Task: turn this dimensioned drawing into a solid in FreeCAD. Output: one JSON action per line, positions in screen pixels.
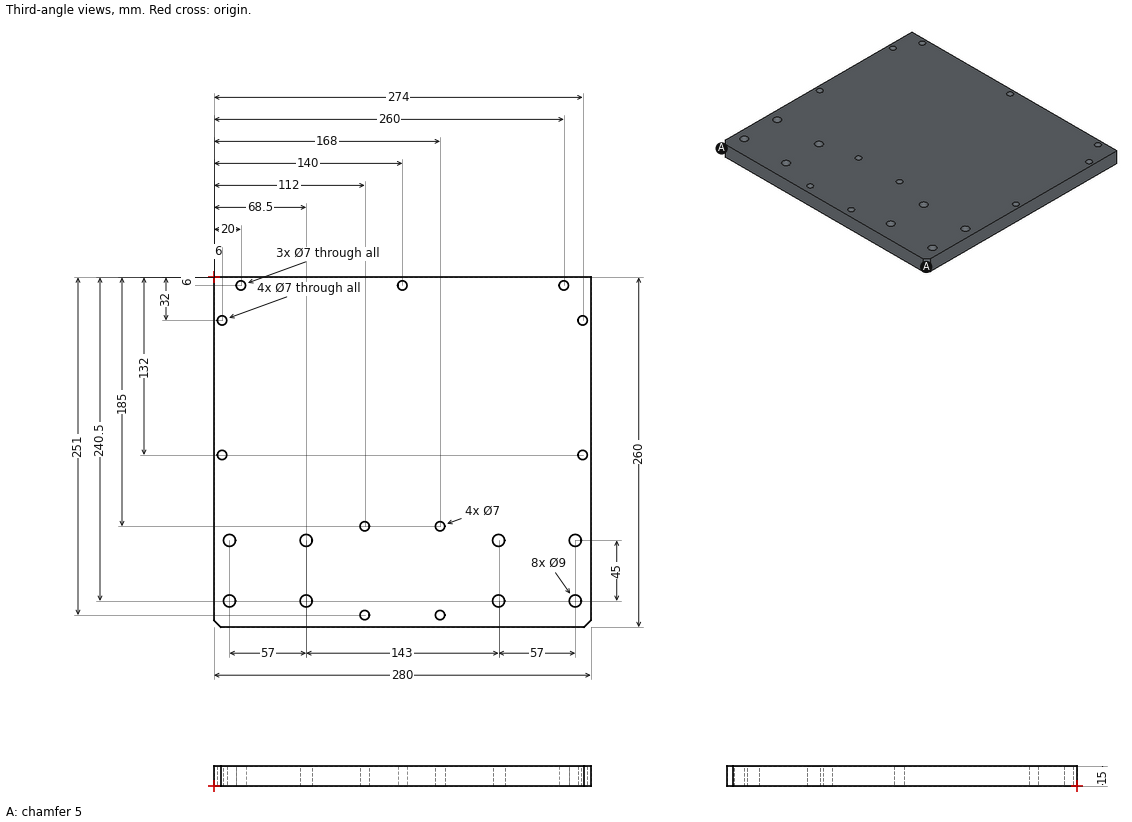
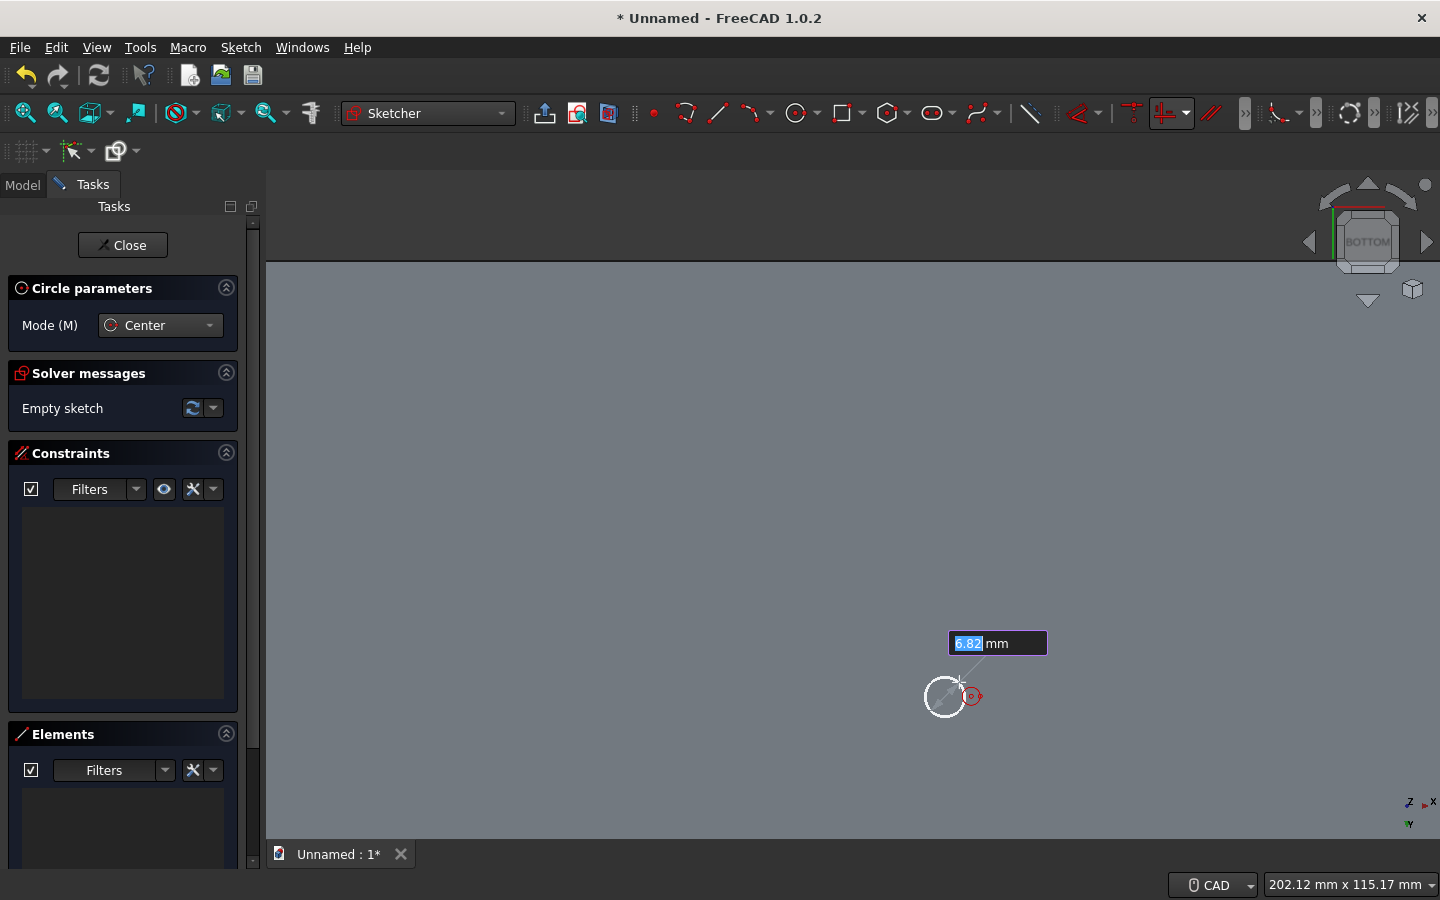
{"action": "type", "text": "7"}
{"action": "key", "text": "Return"}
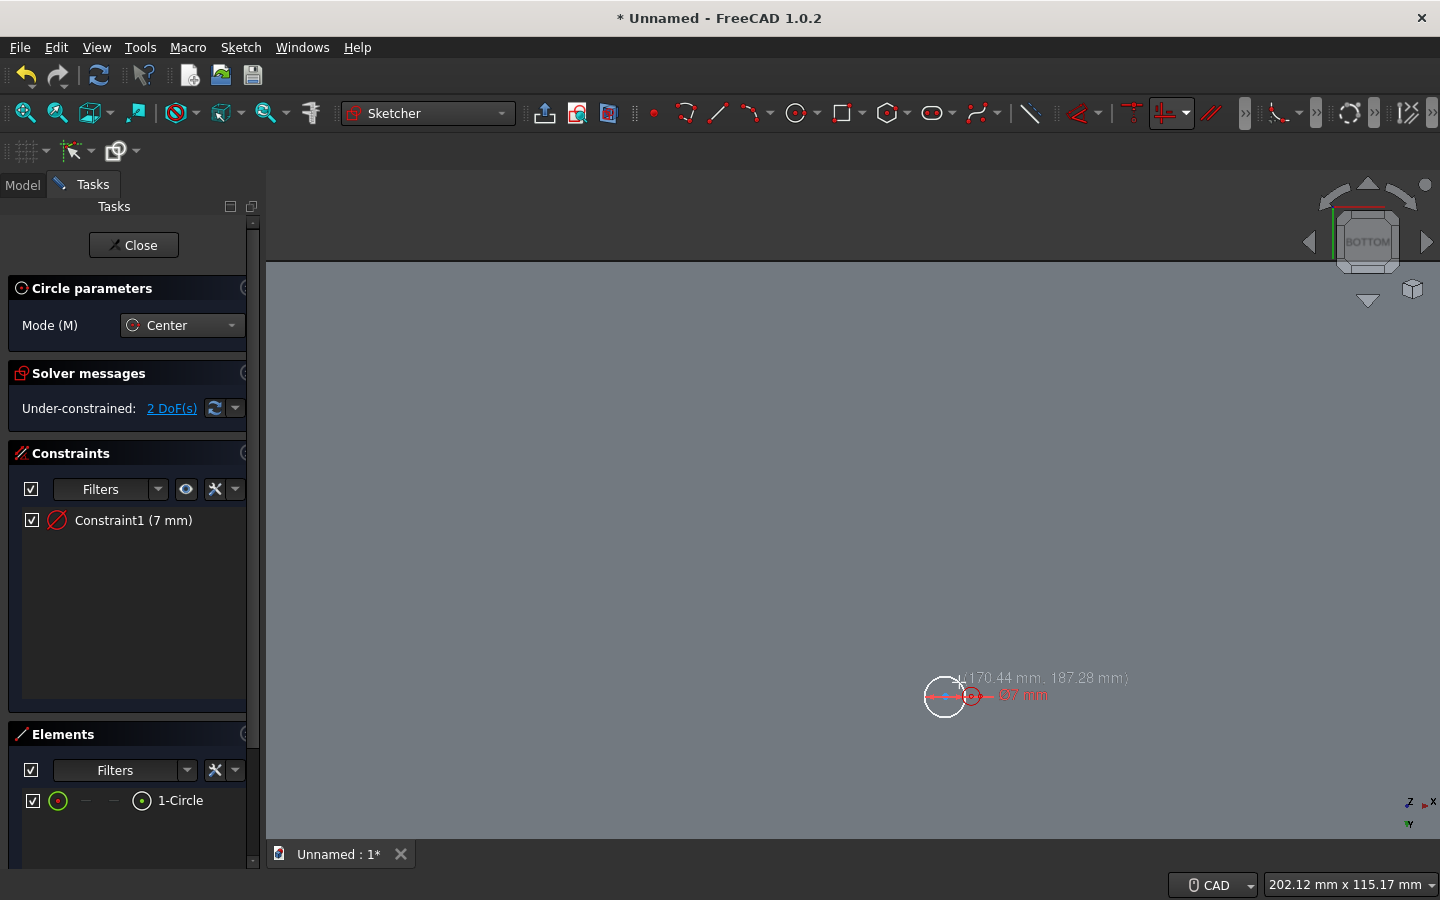
{"action": "left_click", "coordinate": [620, 696]}
{"action": "mouse_move", "coordinate": [634, 682]}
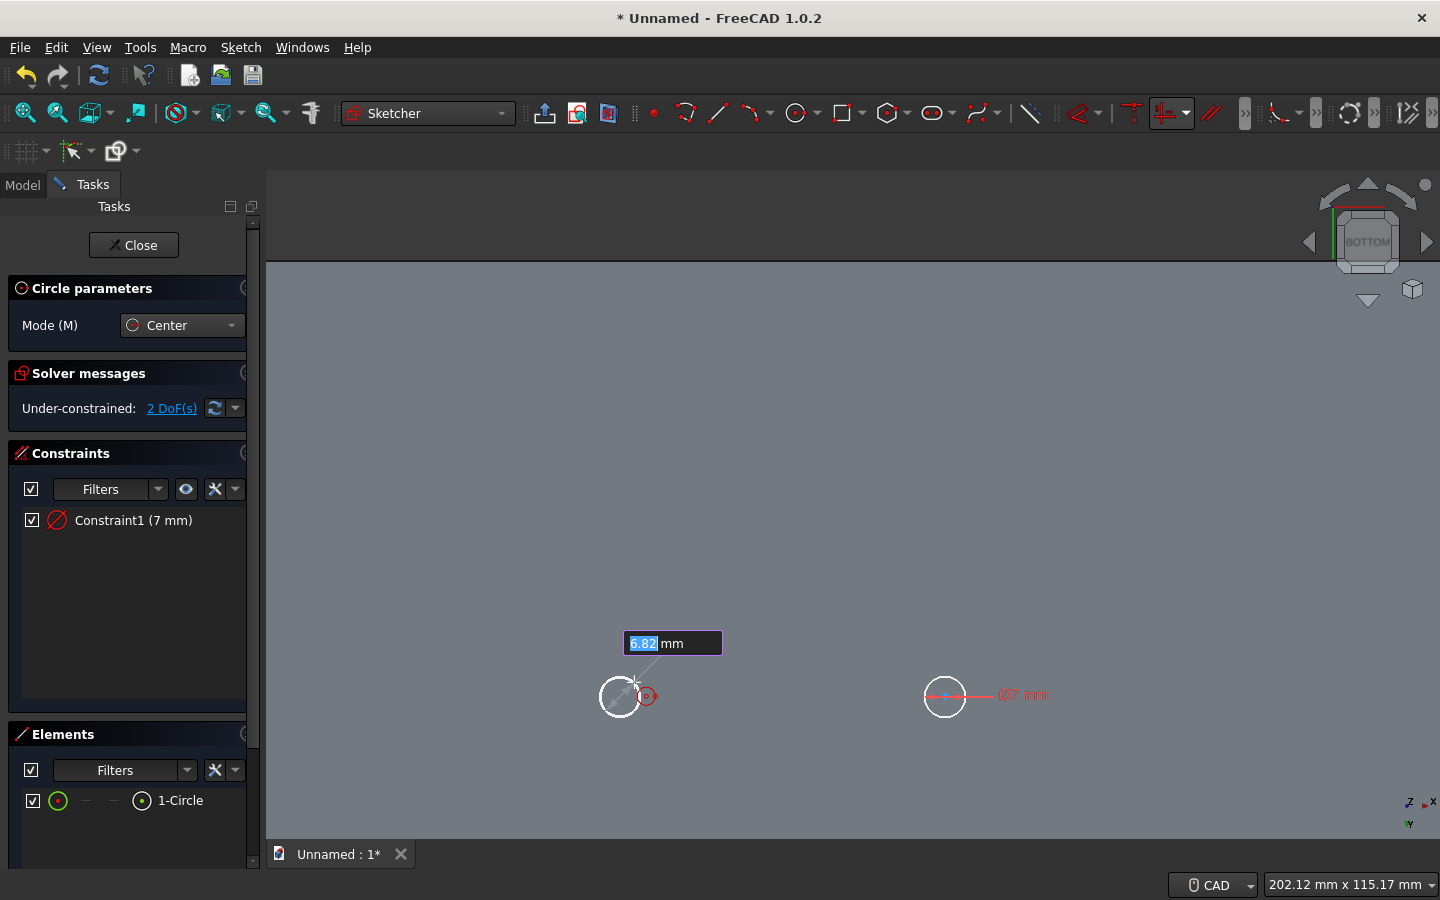
{"action": "type", "text": "7"}
{"action": "key", "text": "Return"}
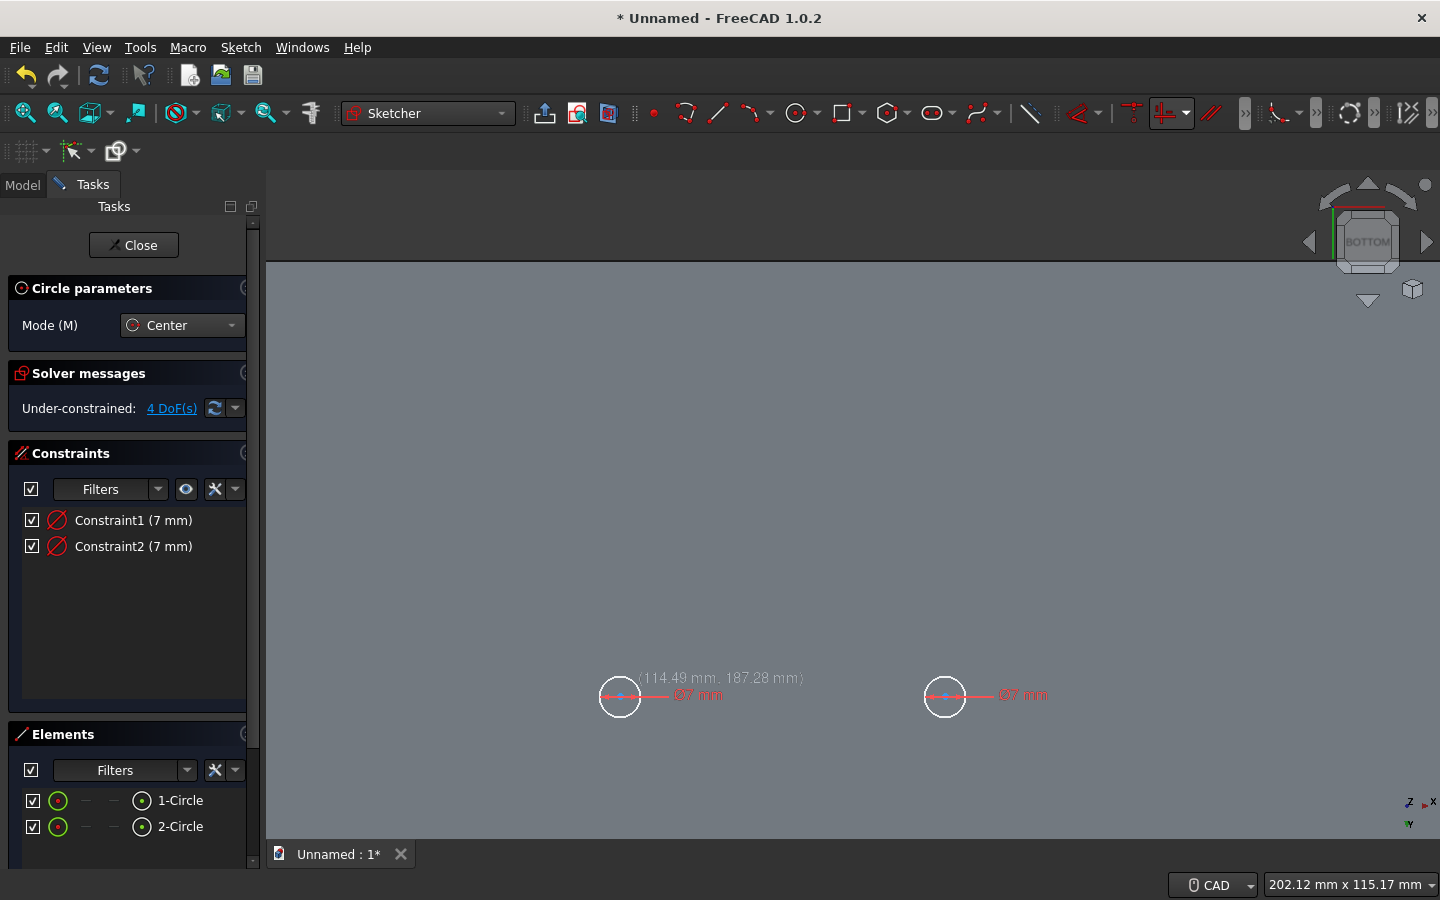
{"action": "left_click", "coordinate": [620, 313]}
{"action": "mouse_move", "coordinate": [634, 298]}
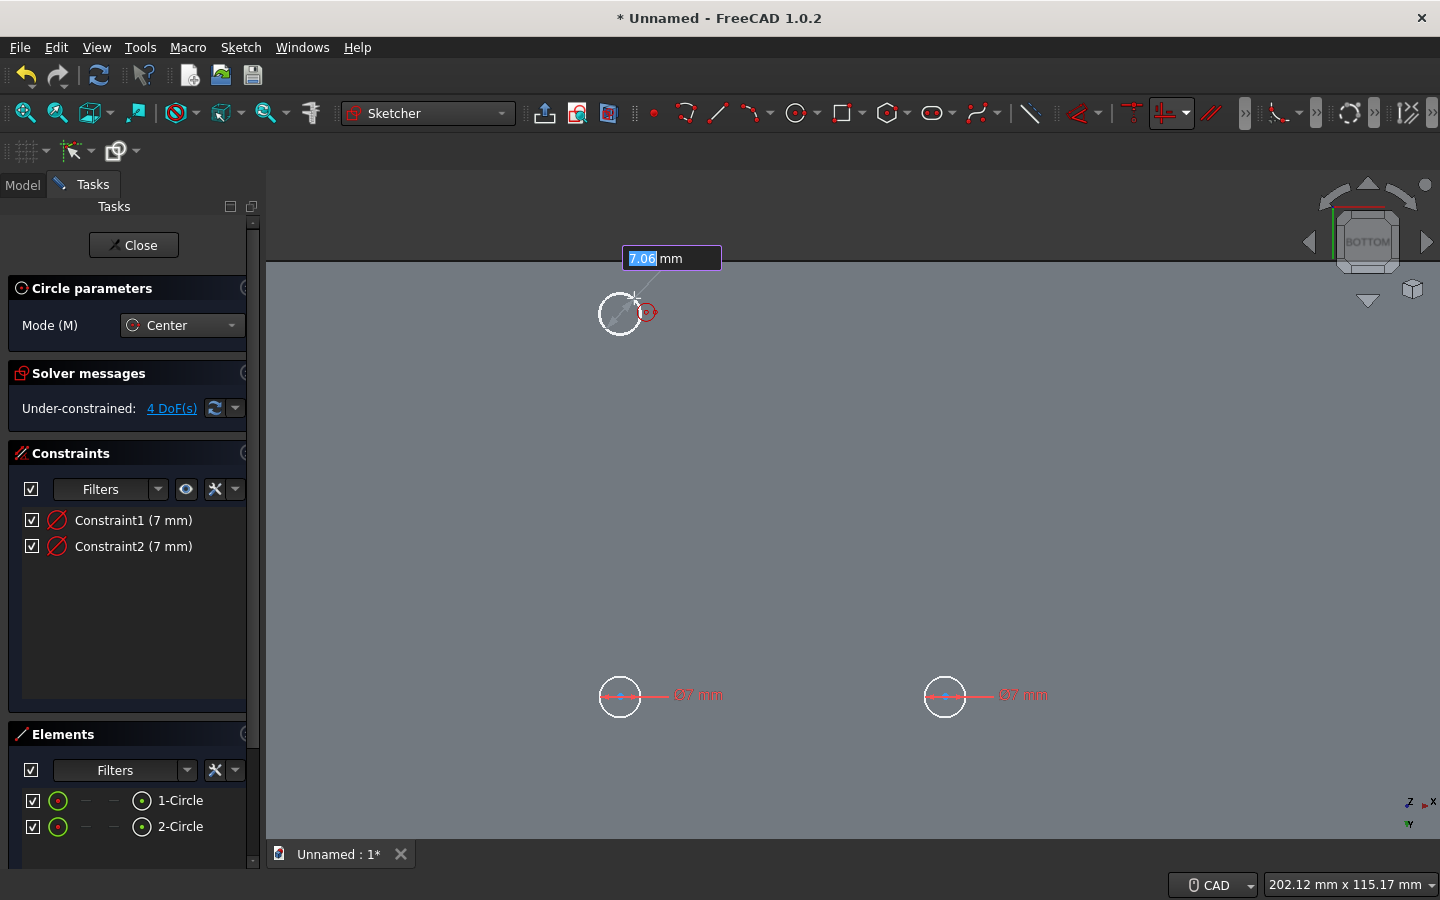
{"action": "type", "text": "7"}
{"action": "key", "text": "Return"}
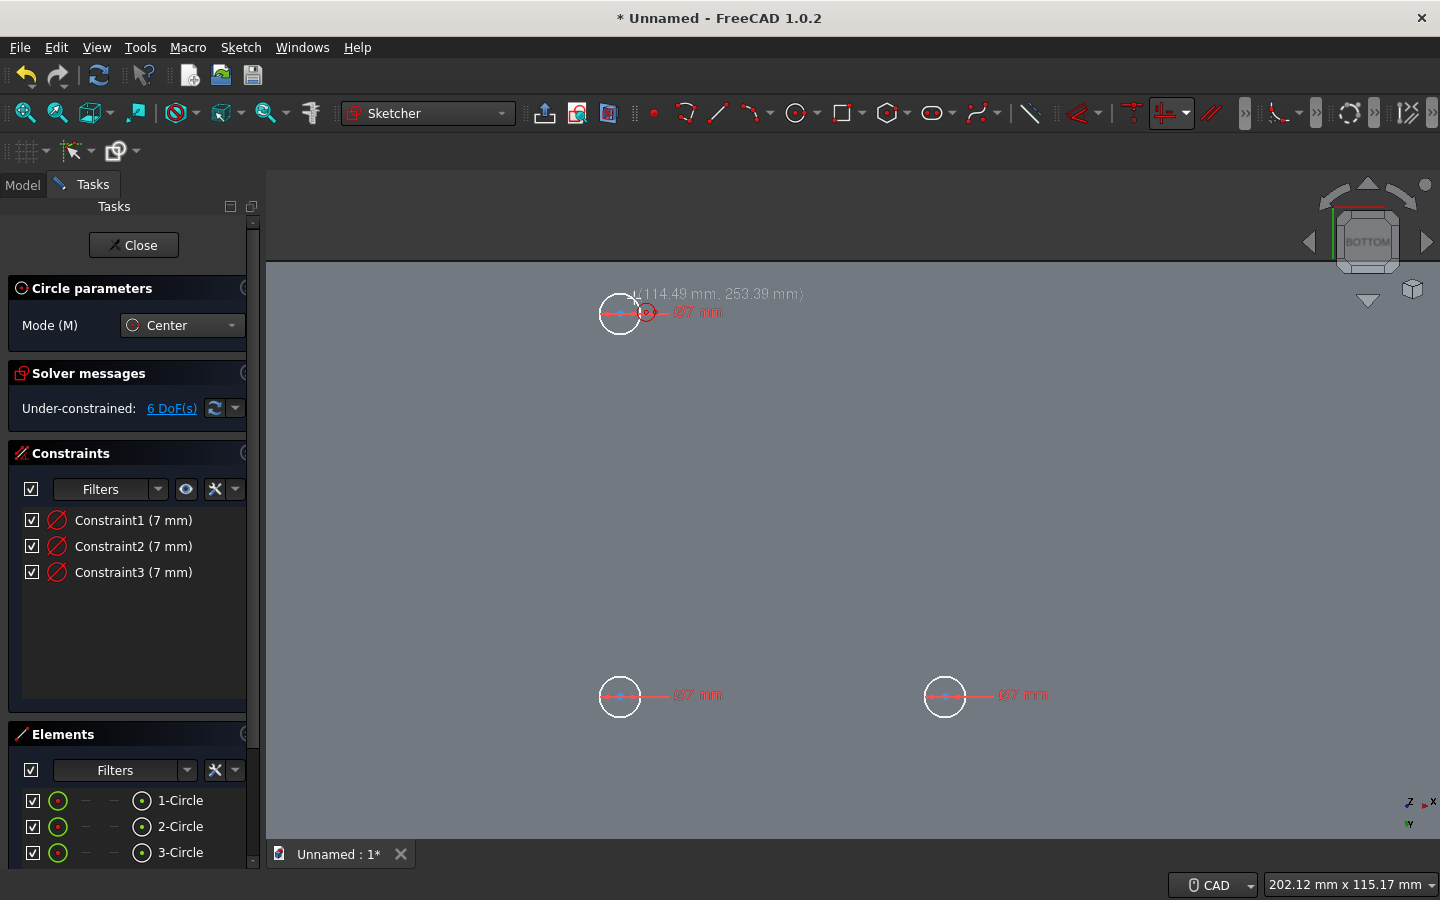
{"action": "left_click", "coordinate": [945, 313]}
{"action": "mouse_move", "coordinate": [959, 298]}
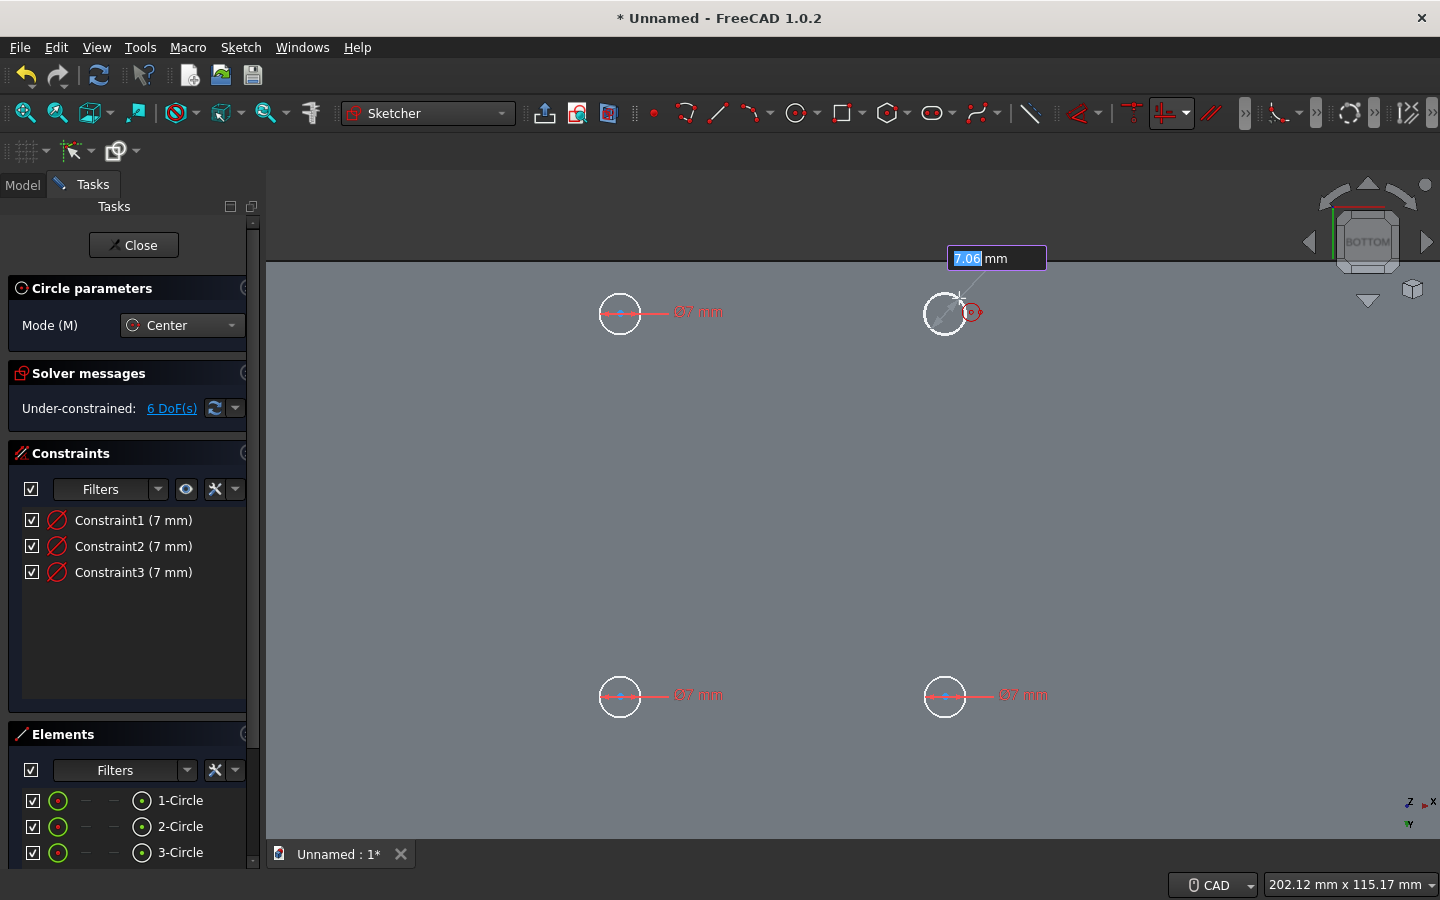
{"action": "type", "text": "7"}
{"action": "key", "text": "Return"}
{"action": "key", "text": "Escape"}